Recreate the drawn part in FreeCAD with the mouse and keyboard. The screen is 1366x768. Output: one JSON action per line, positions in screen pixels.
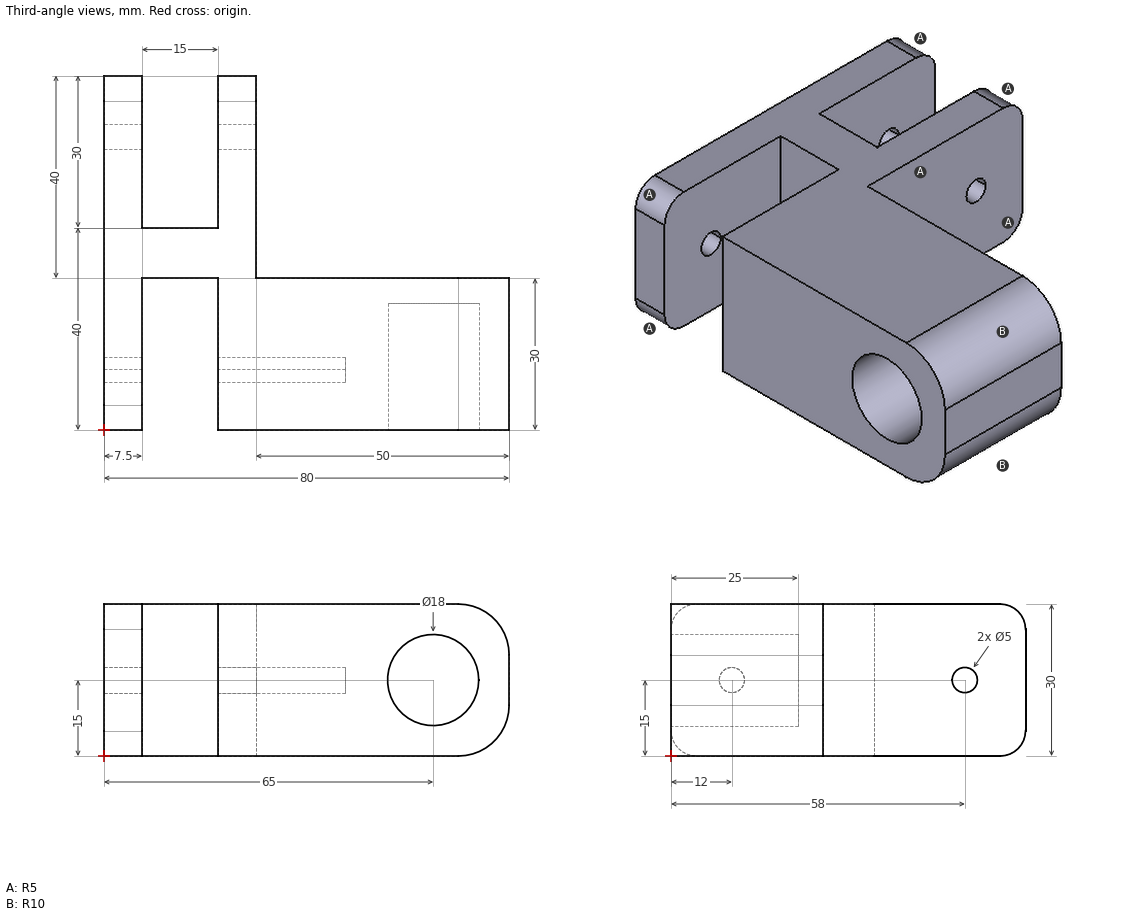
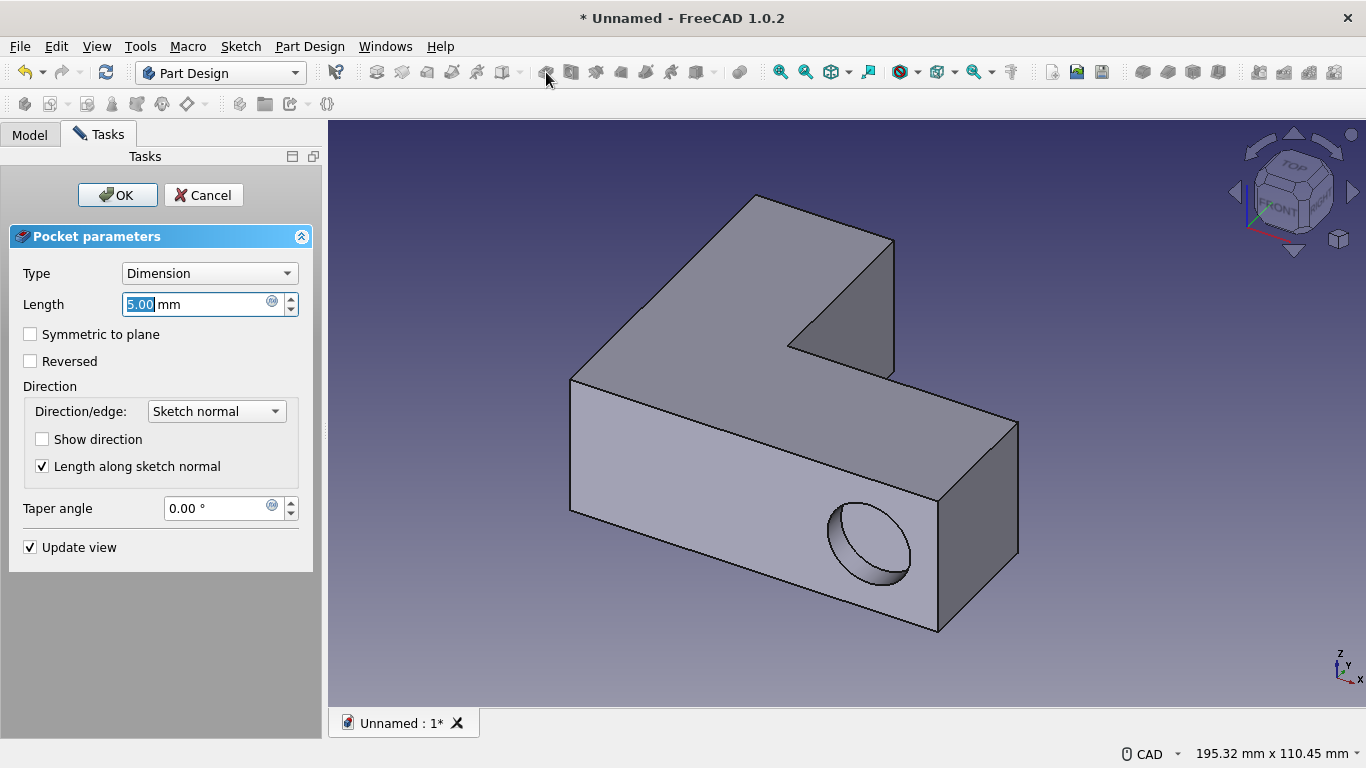
{"action": "type", "text": "25"}
{"action": "key", "text": "Tab"}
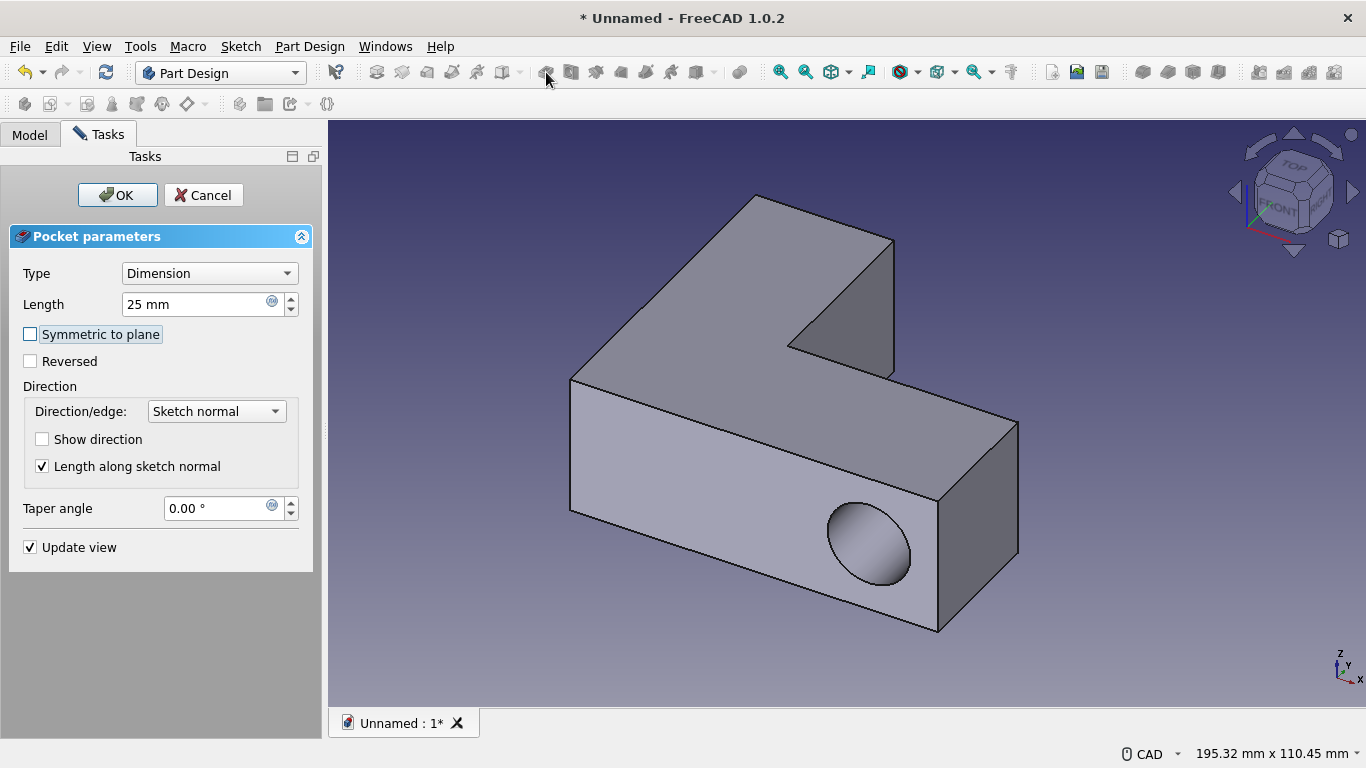
{"action": "left_click", "coordinate": [118, 195]}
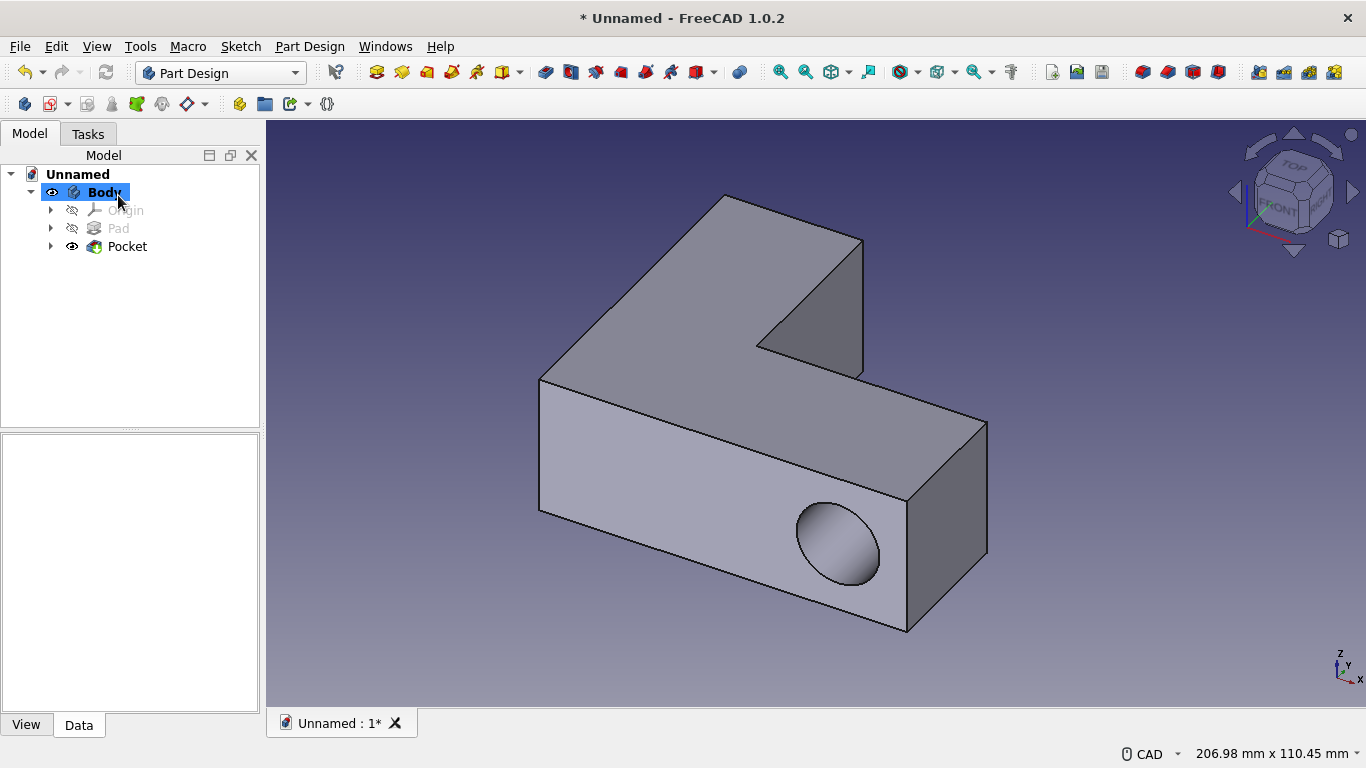
{"action": "key", "text": "5"}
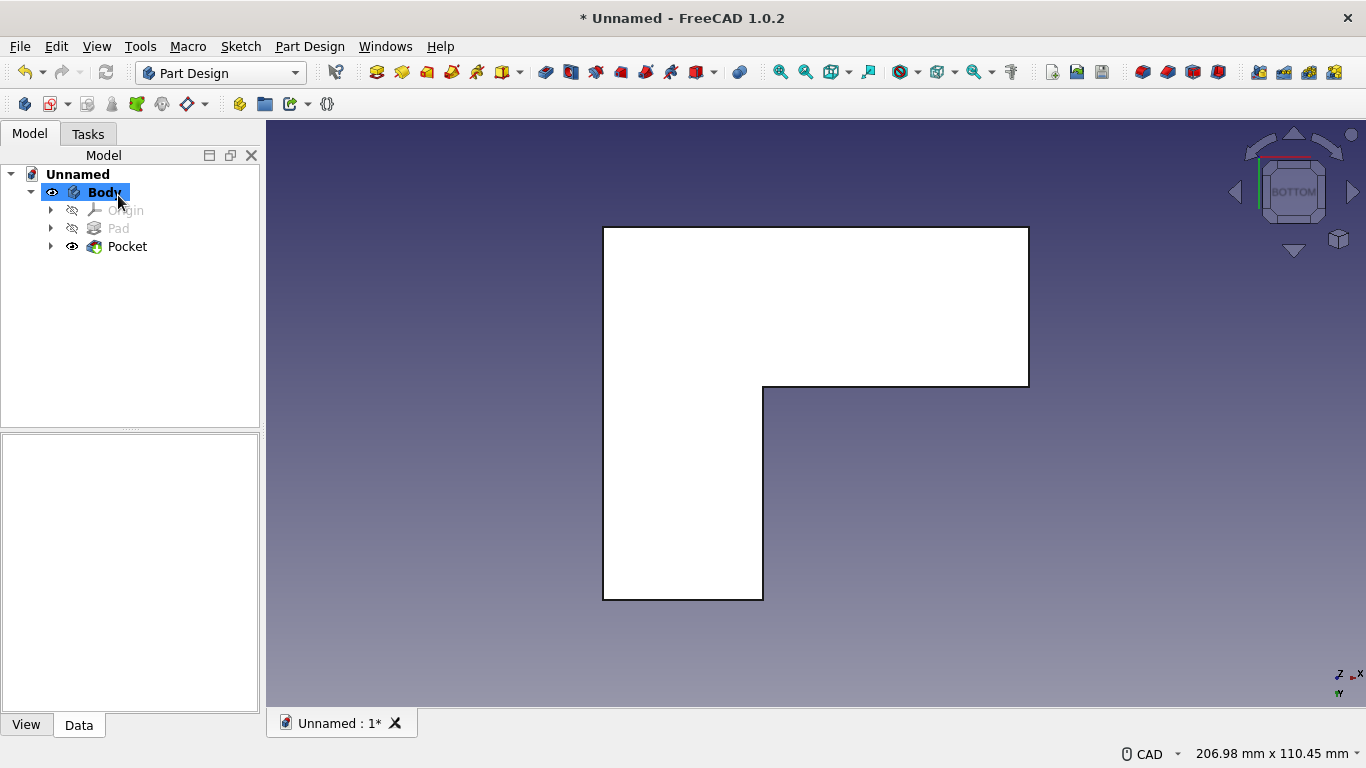
{"action": "left_click", "coordinate": [937, 306]}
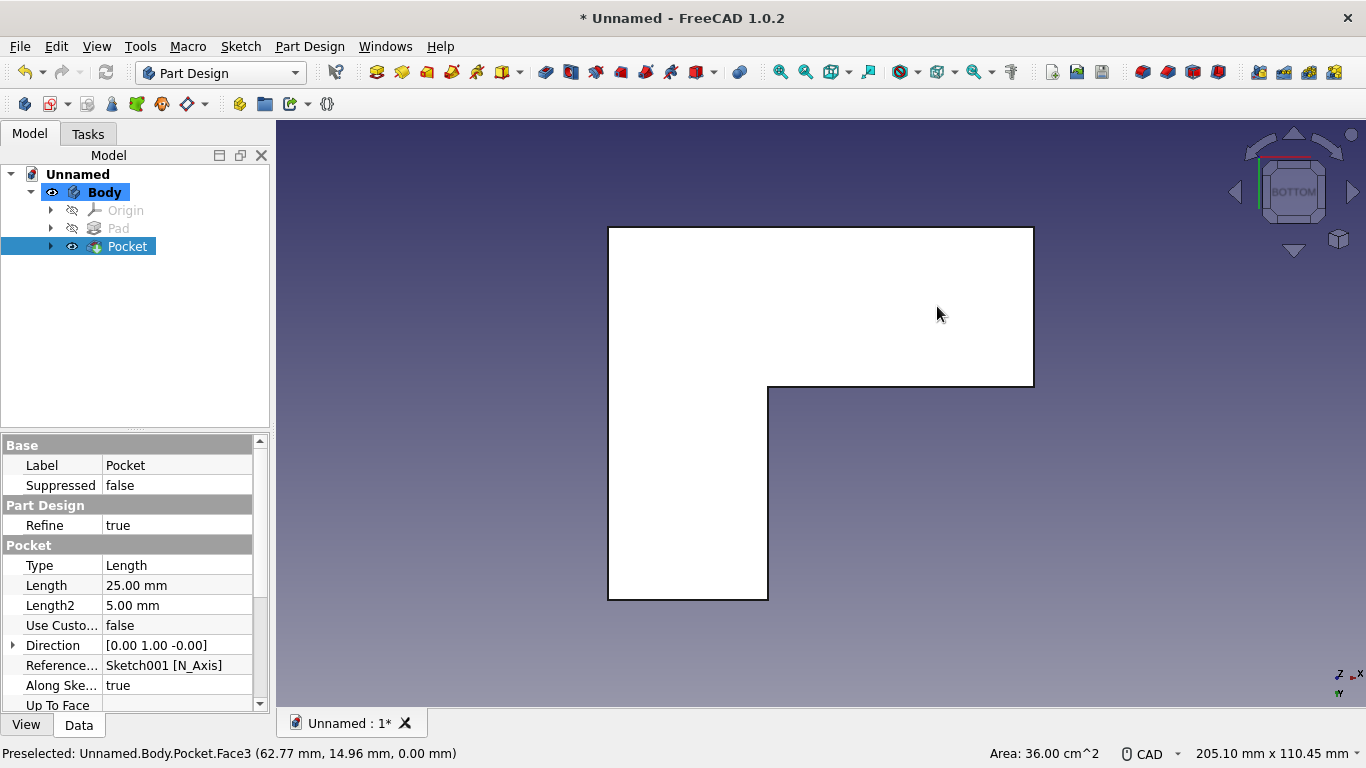
{"action": "left_click", "coordinate": [50, 104]}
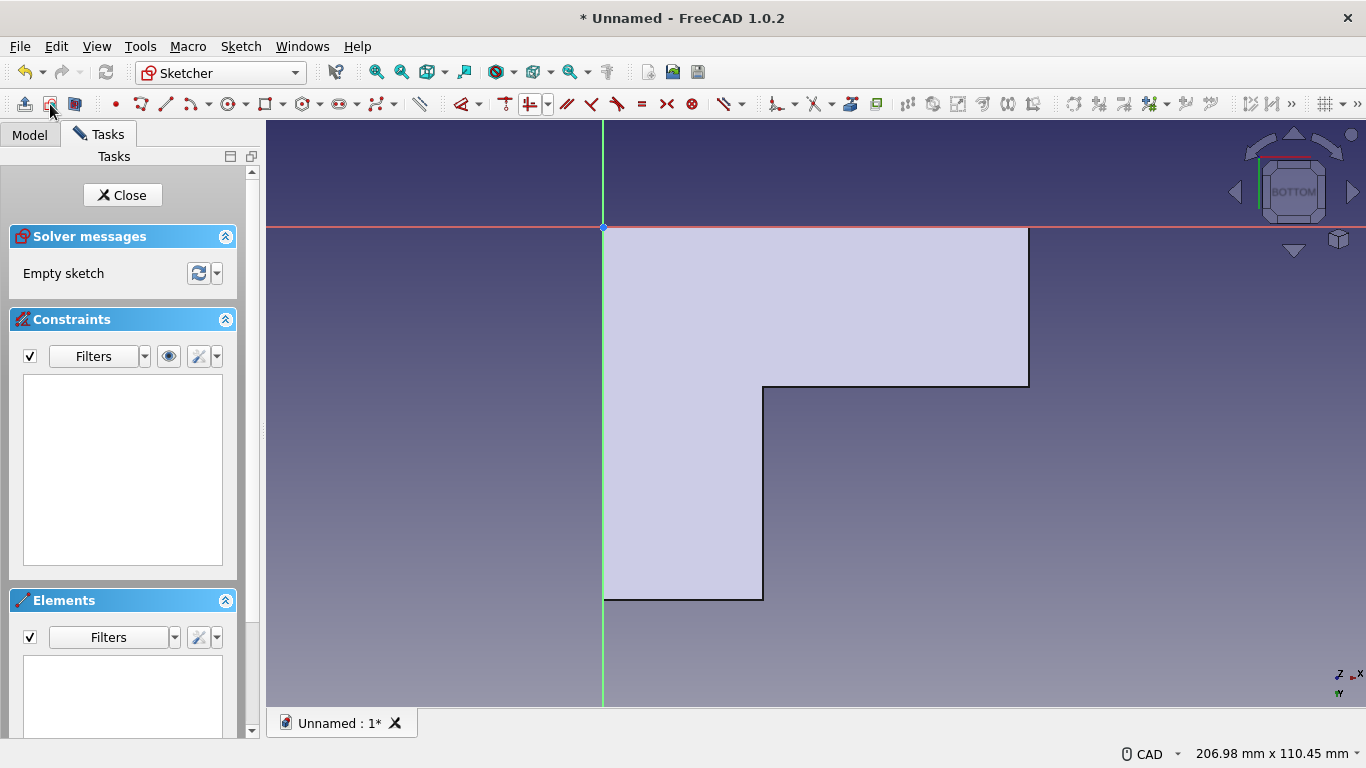
{"action": "key", "text": "g r"}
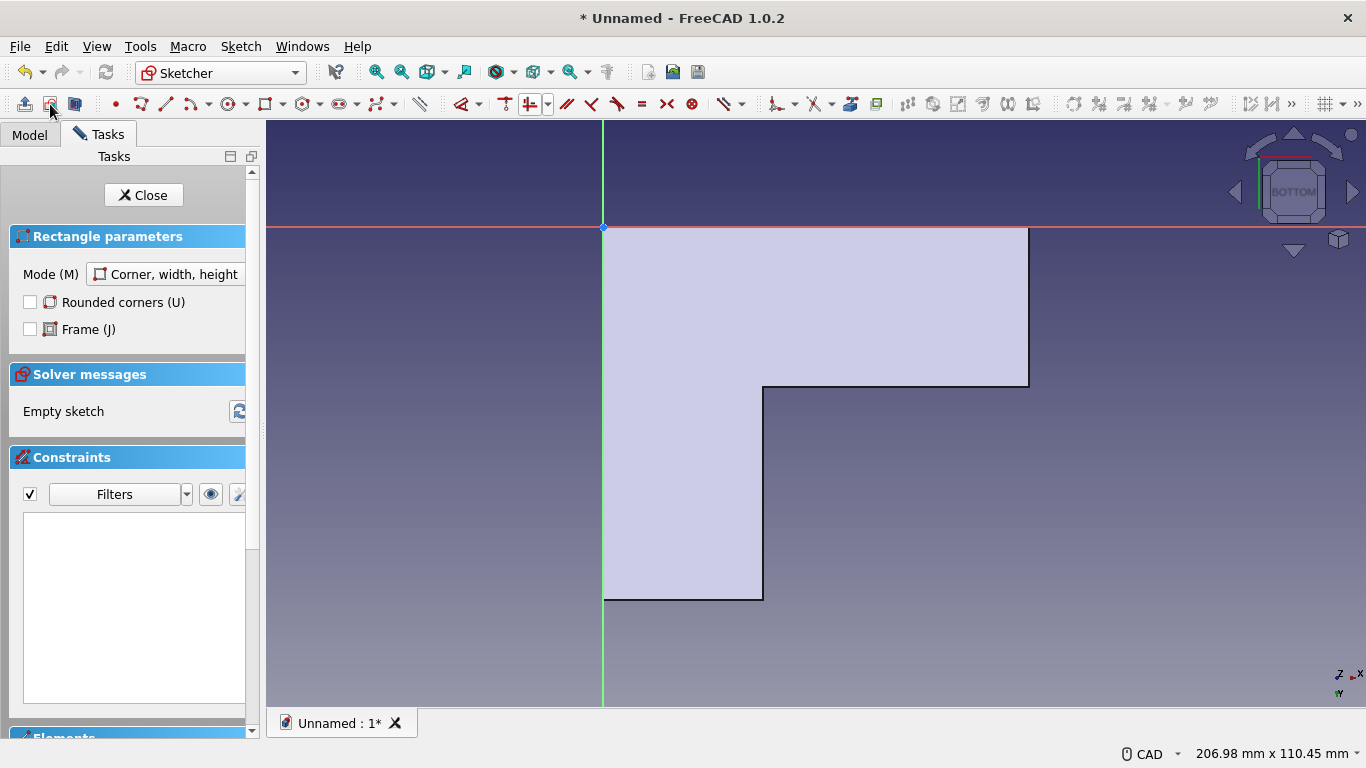
{"action": "left_click", "coordinate": [643, 440]}
{"action": "left_click", "coordinate": [723, 600]}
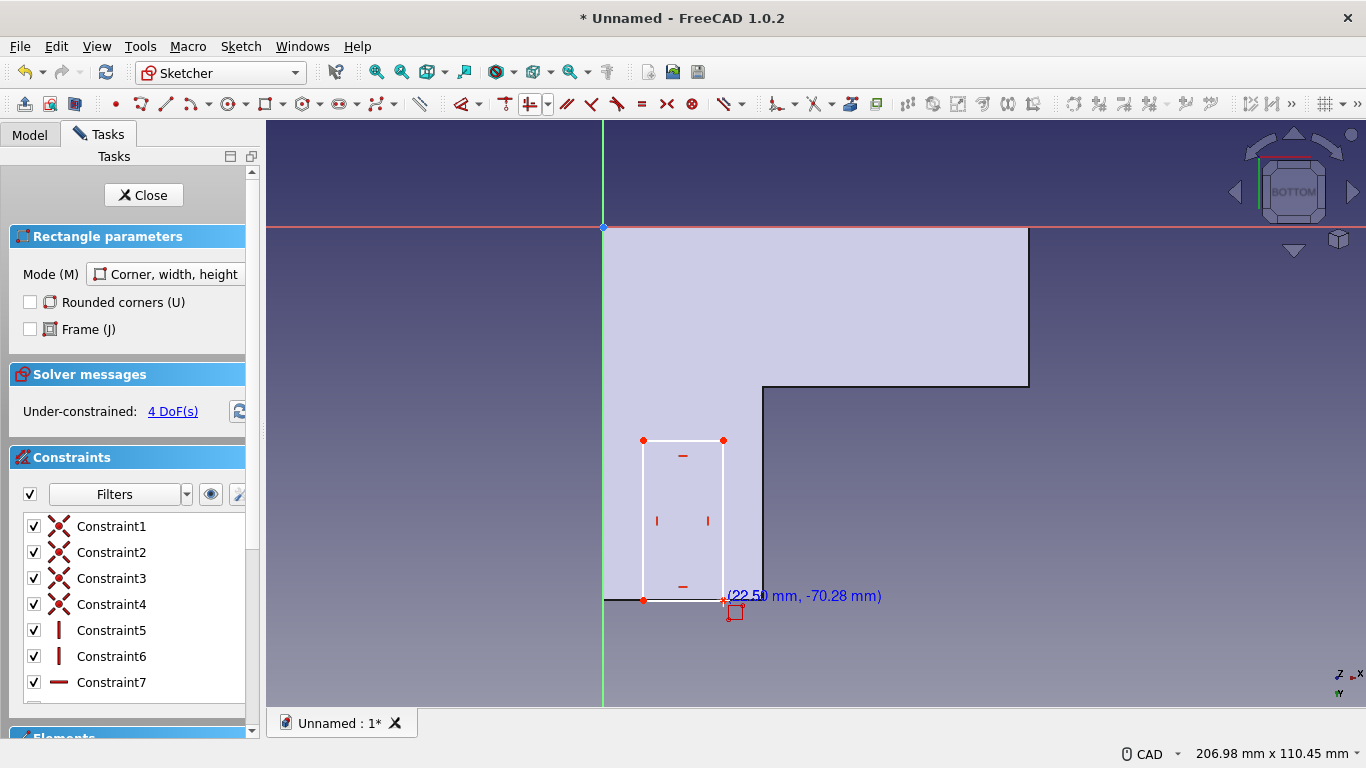
{"action": "left_click", "coordinate": [643, 227]}
{"action": "left_click", "coordinate": [723, 387]}
{"action": "key", "text": "Escape"}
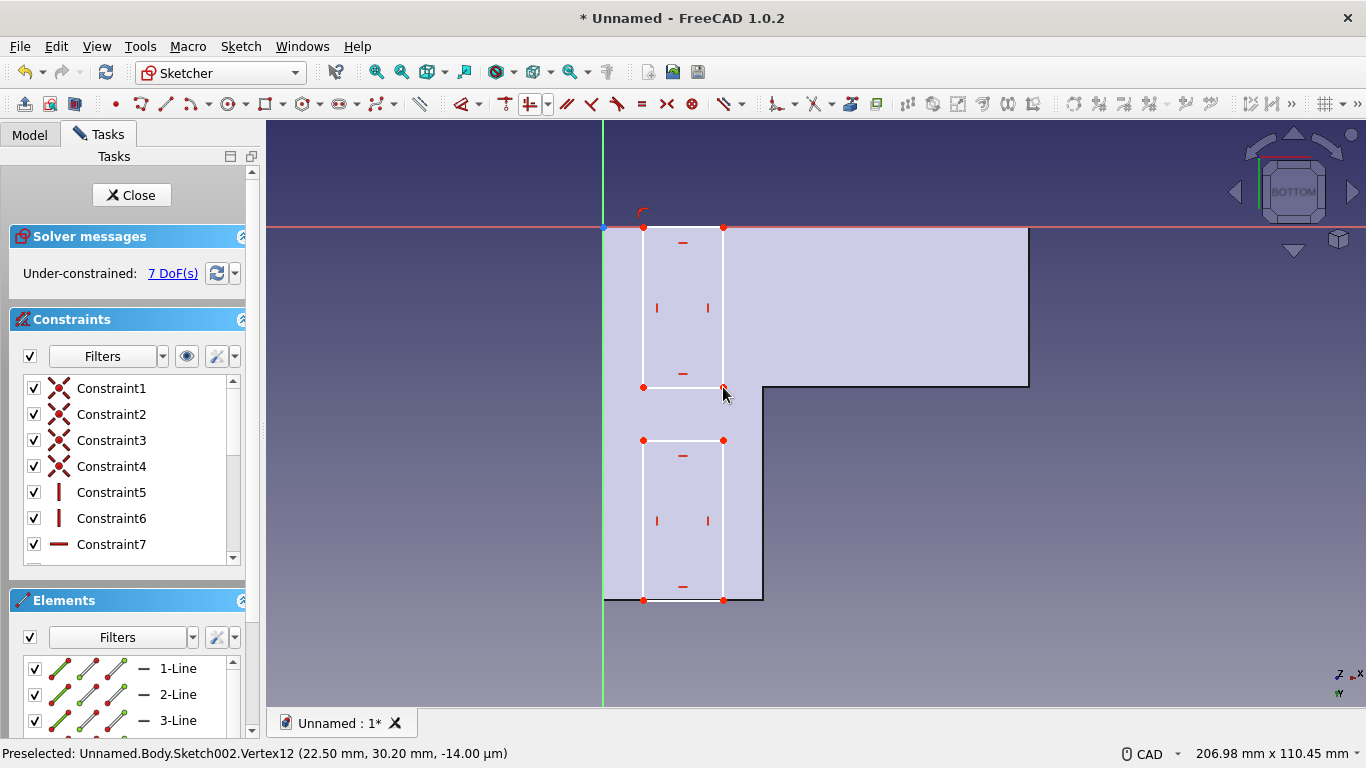
{"action": "left_click", "coordinate": [460, 104]}